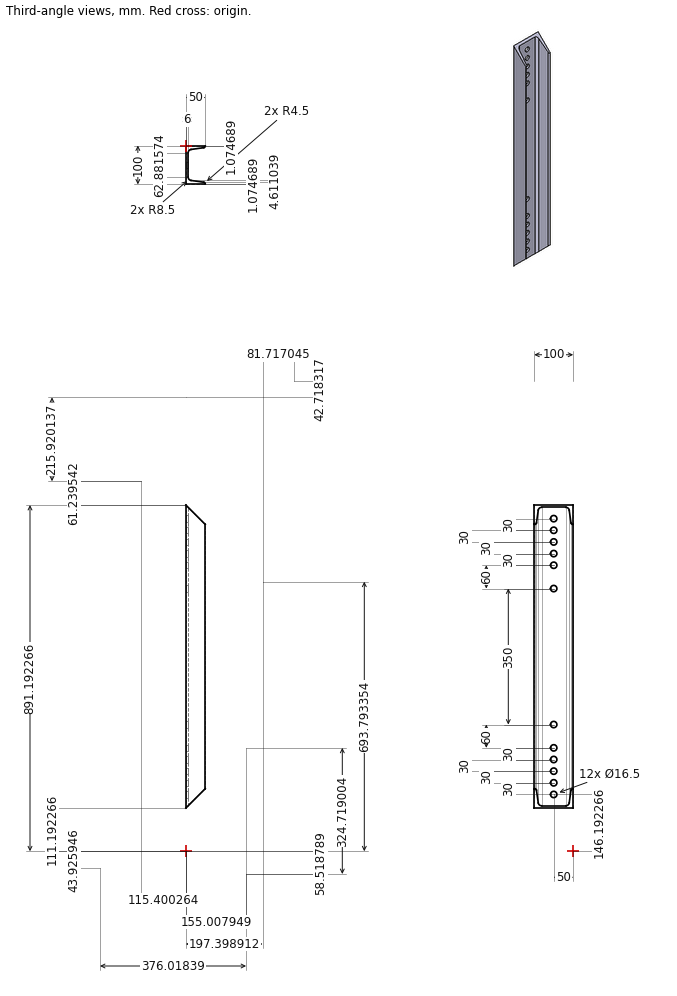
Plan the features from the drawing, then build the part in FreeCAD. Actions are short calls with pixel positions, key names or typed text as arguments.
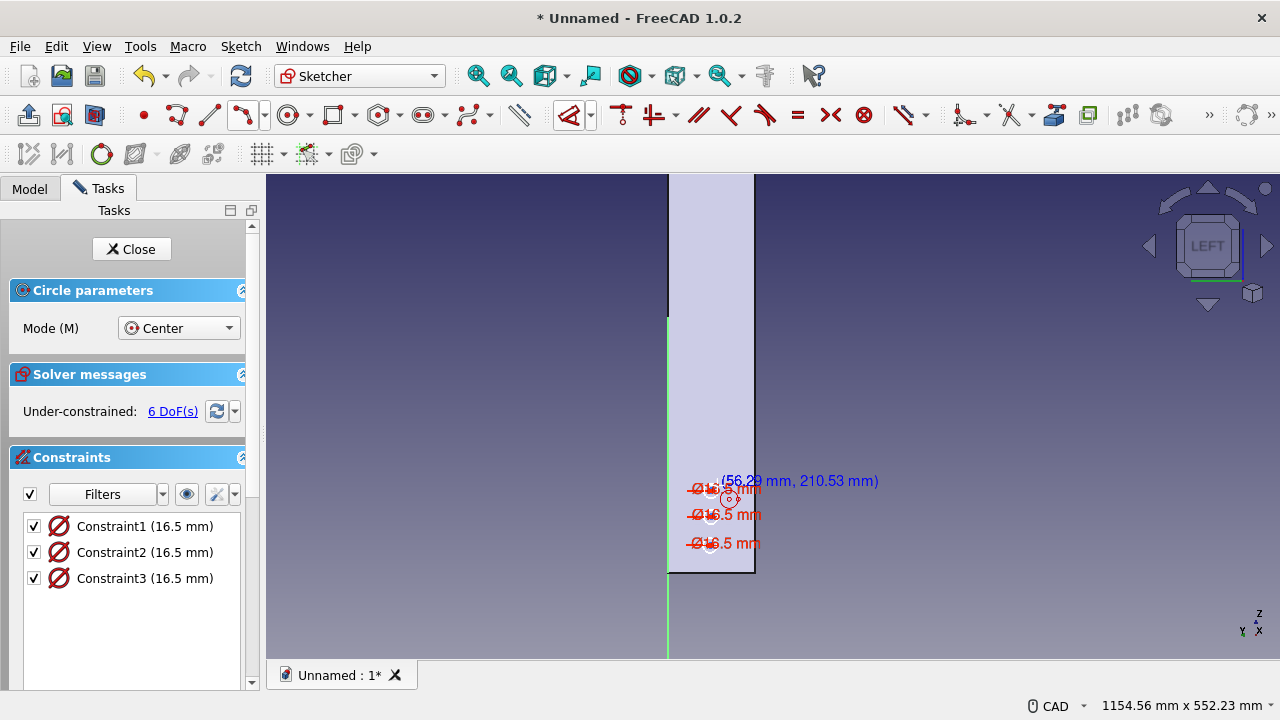
scroll(711, 463, up, 6)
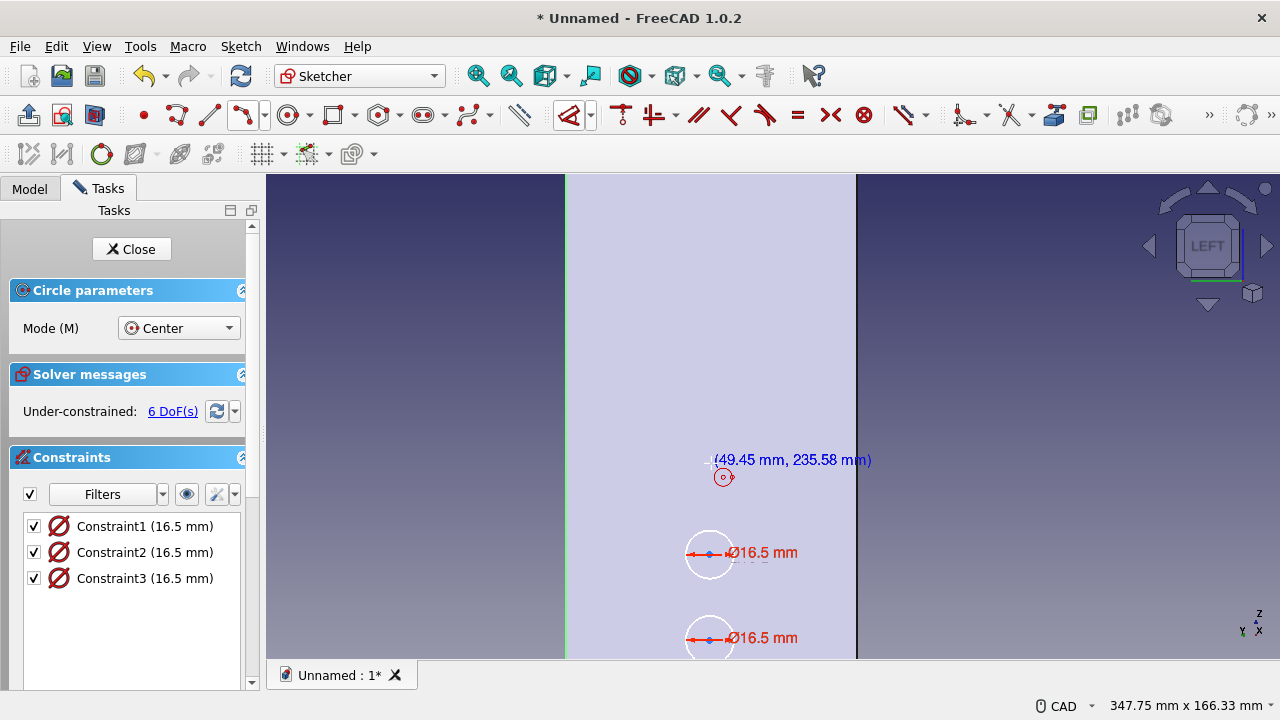
scroll(711, 482, down, 11)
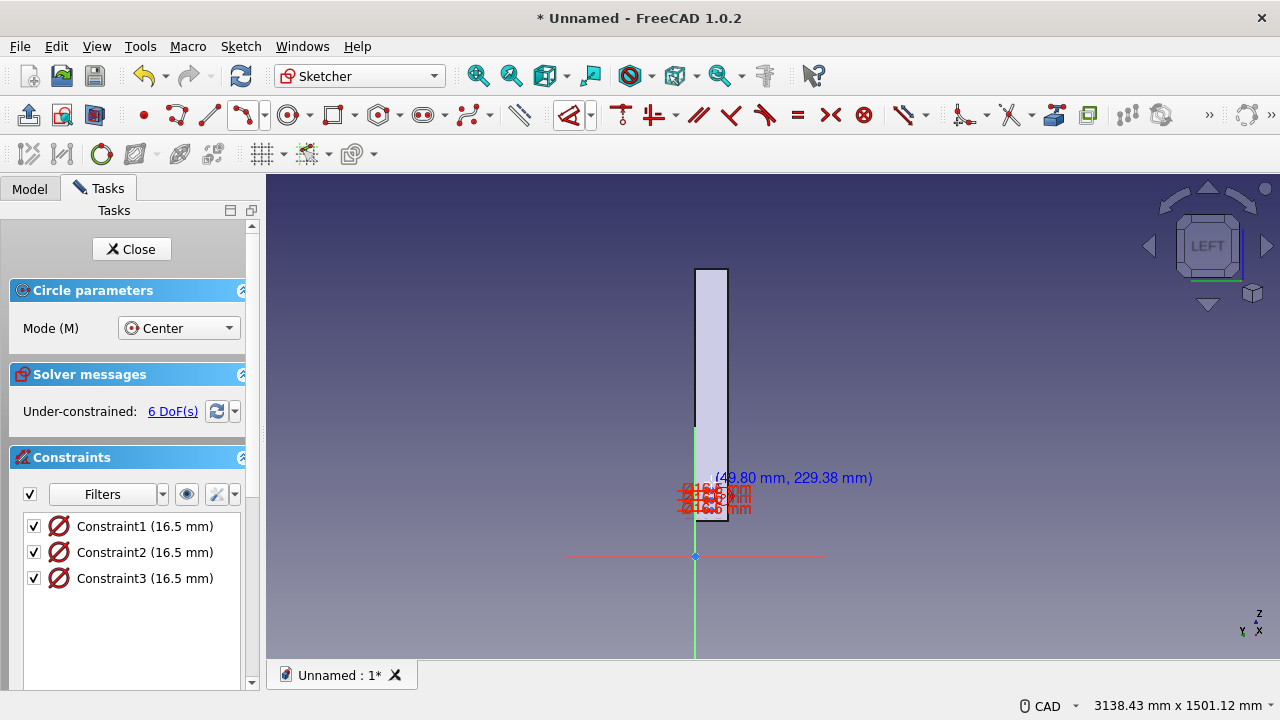
scroll(711, 480, up, 5)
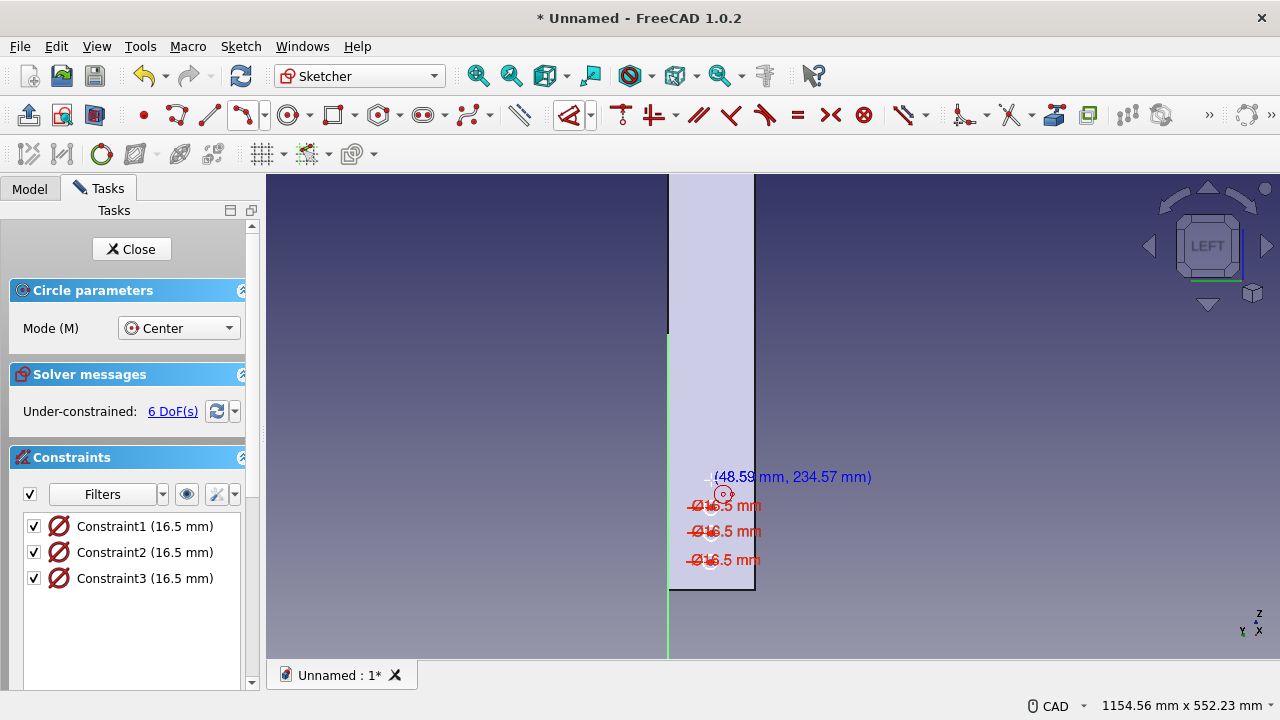
click(711, 480)
move(717, 475)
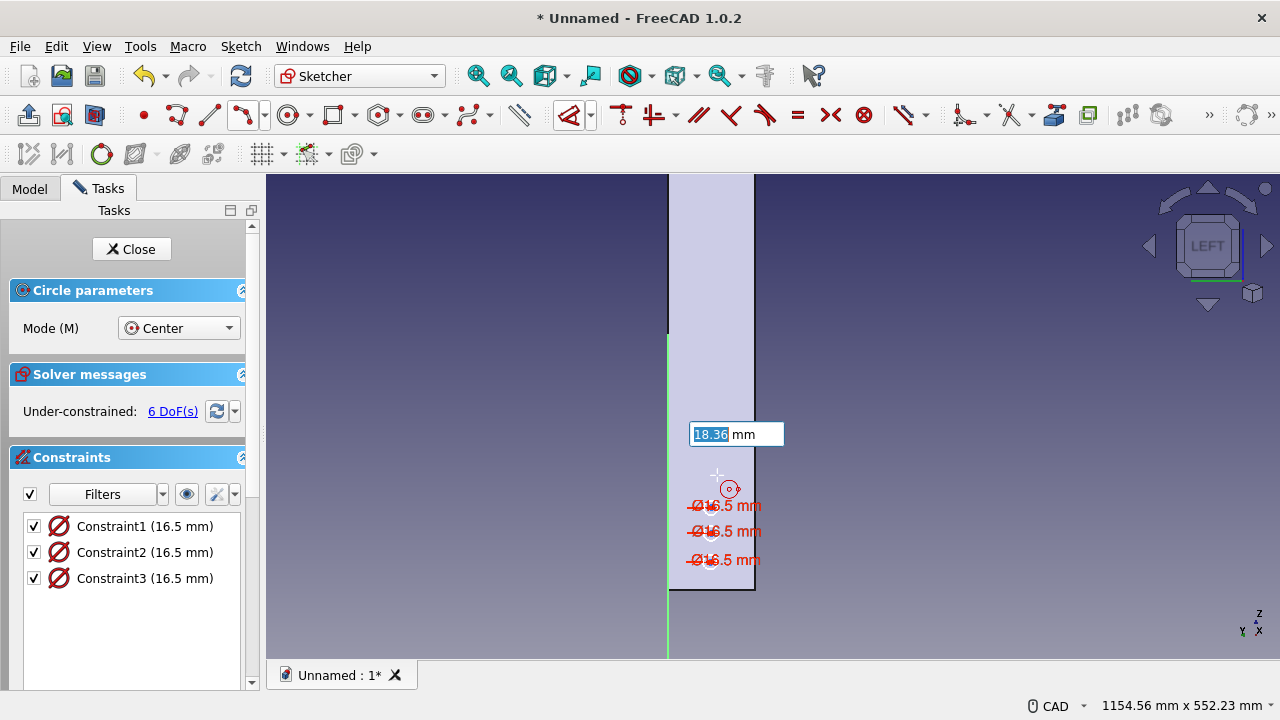
text(16.5)
key(Return)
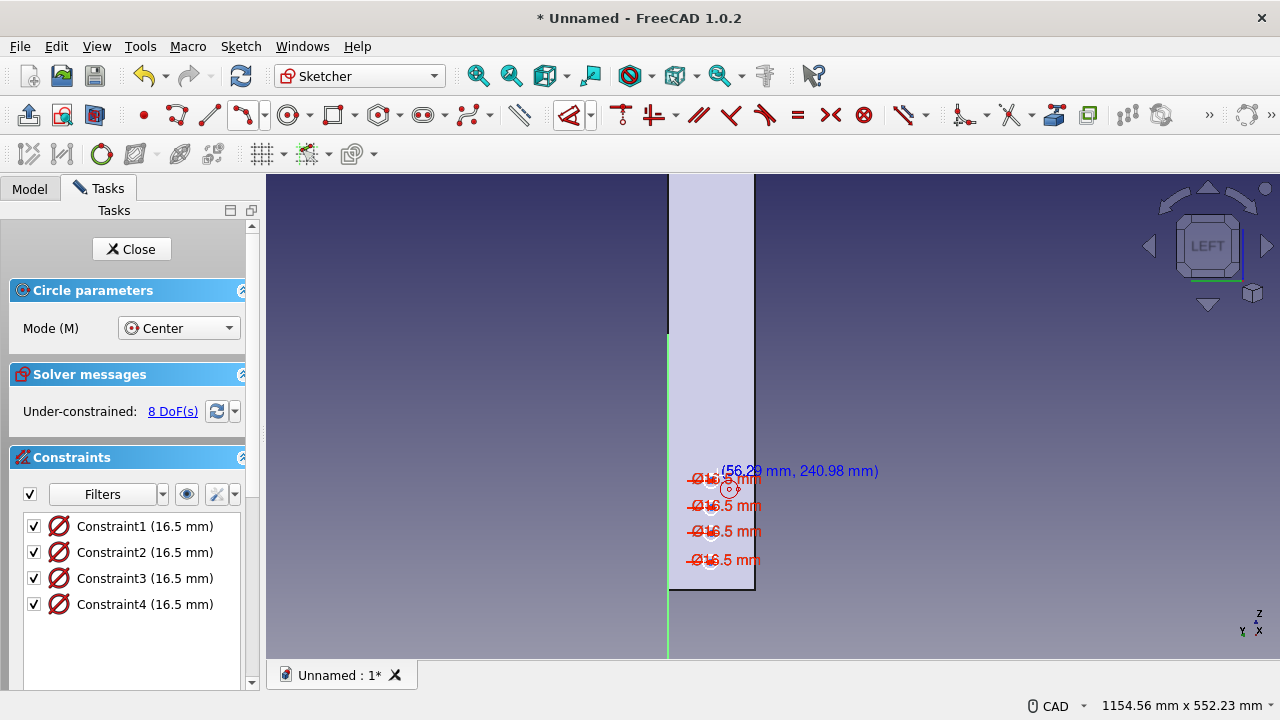
scroll(711, 454, up, 6)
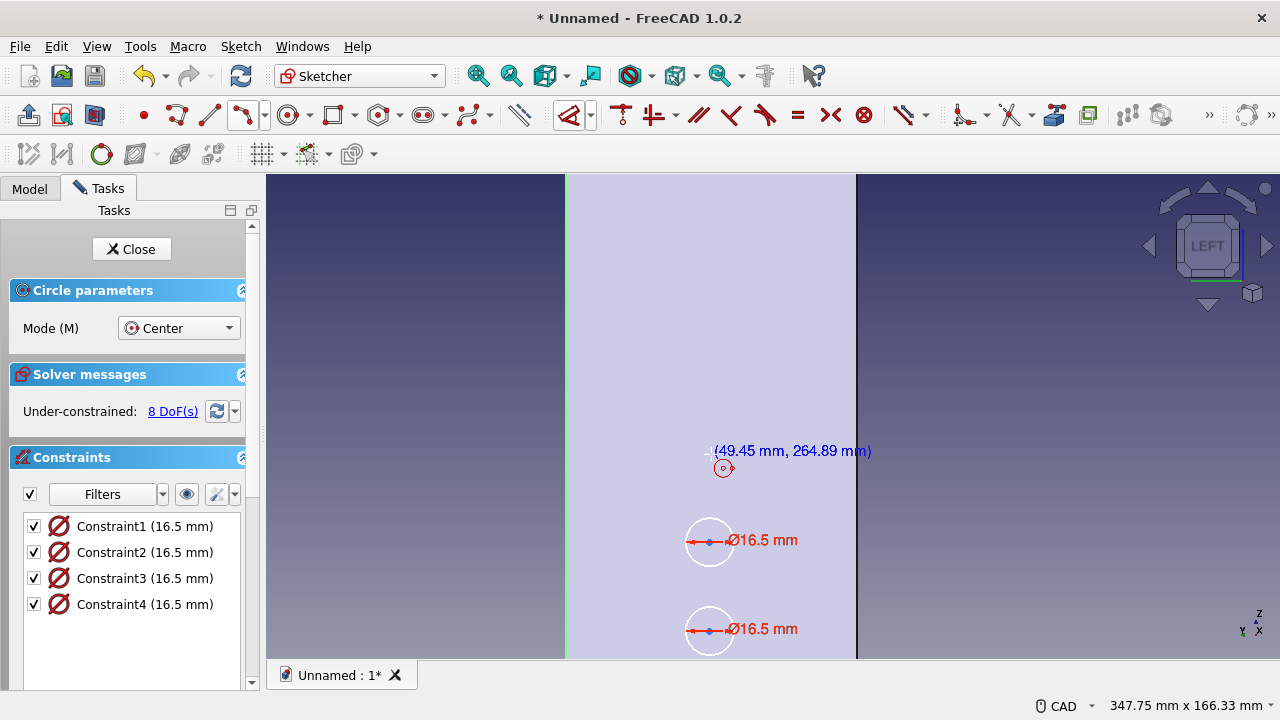
scroll(711, 472, down, 11)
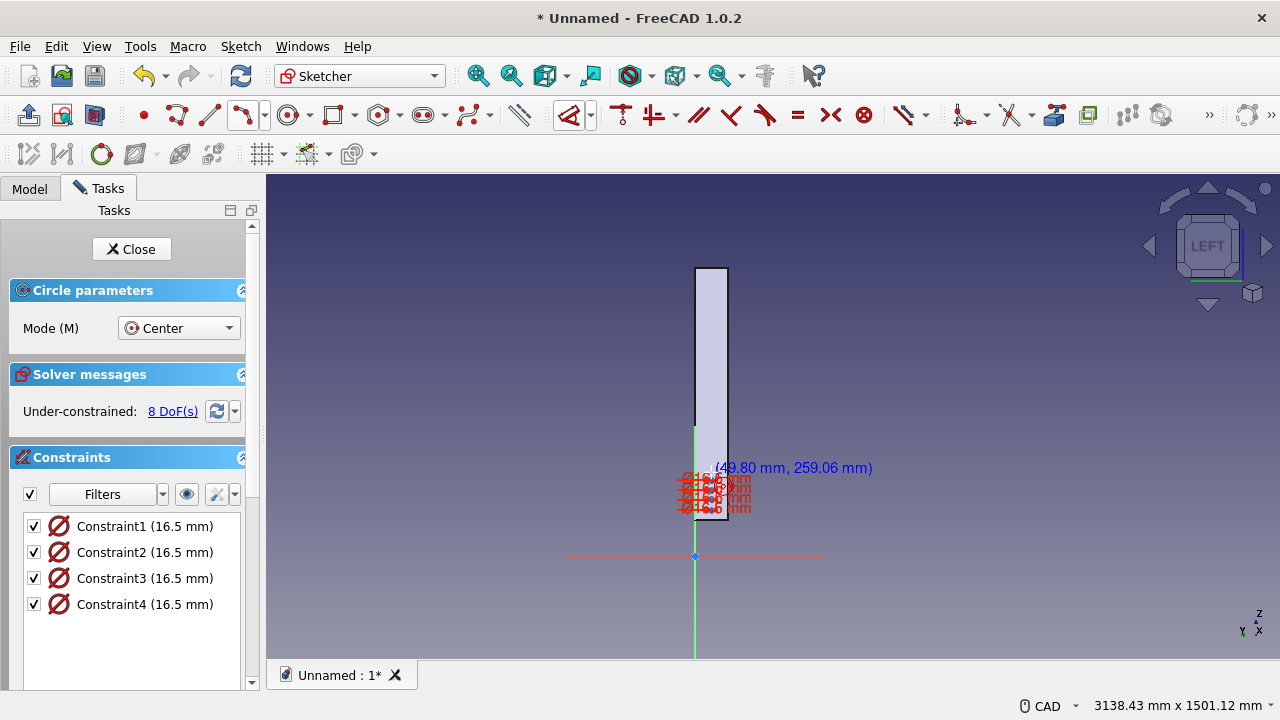
scroll(711, 470, up, 5)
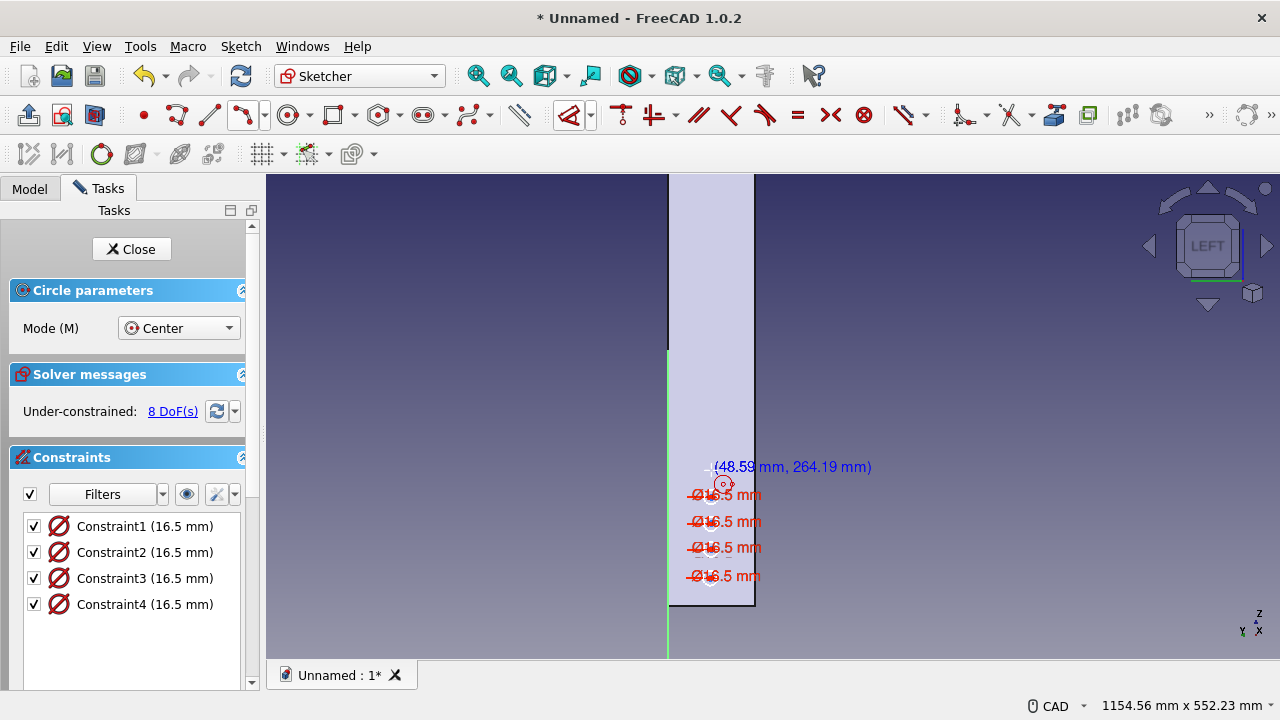
click(711, 470)
move(717, 465)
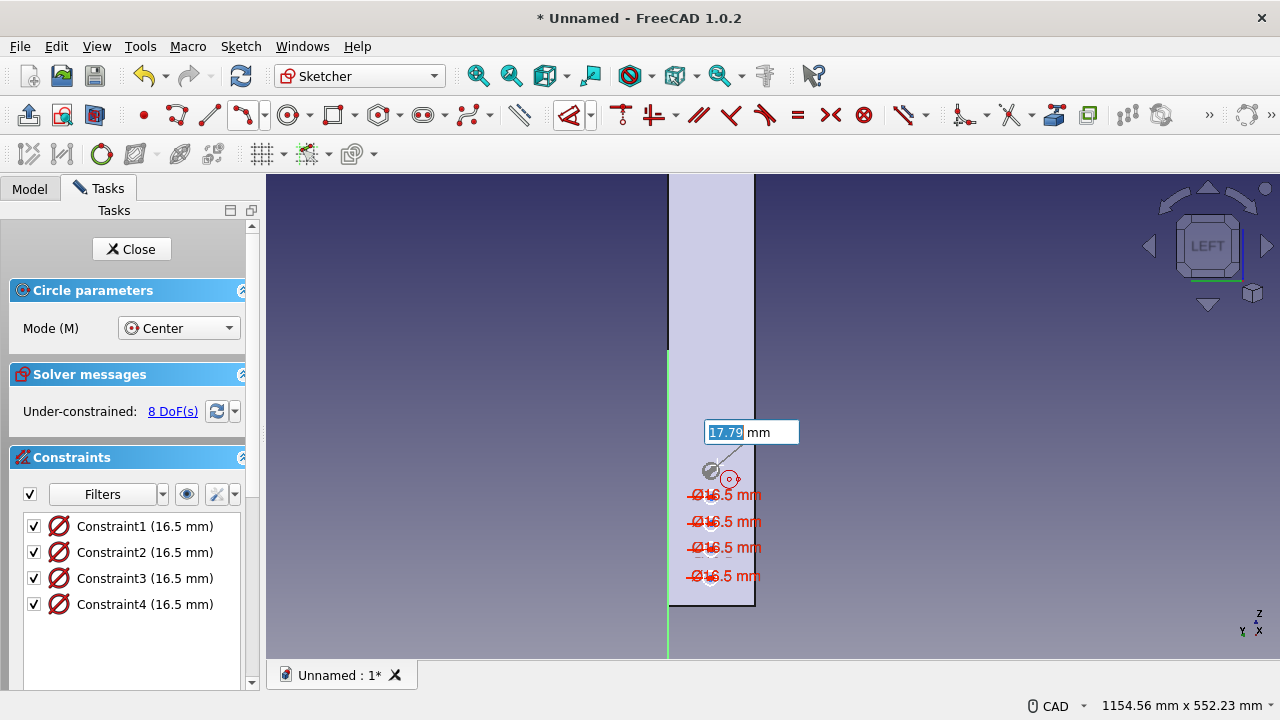
text(16.5)
key(Return)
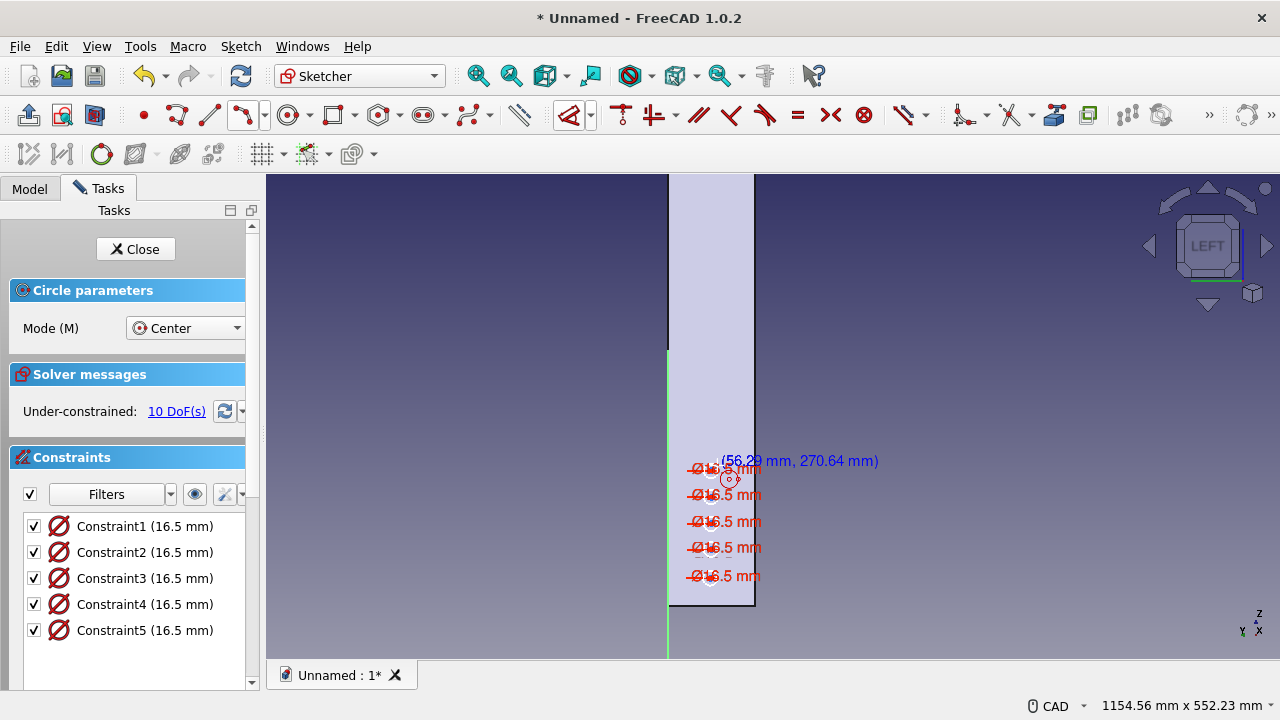
scroll(711, 417, up, 6)